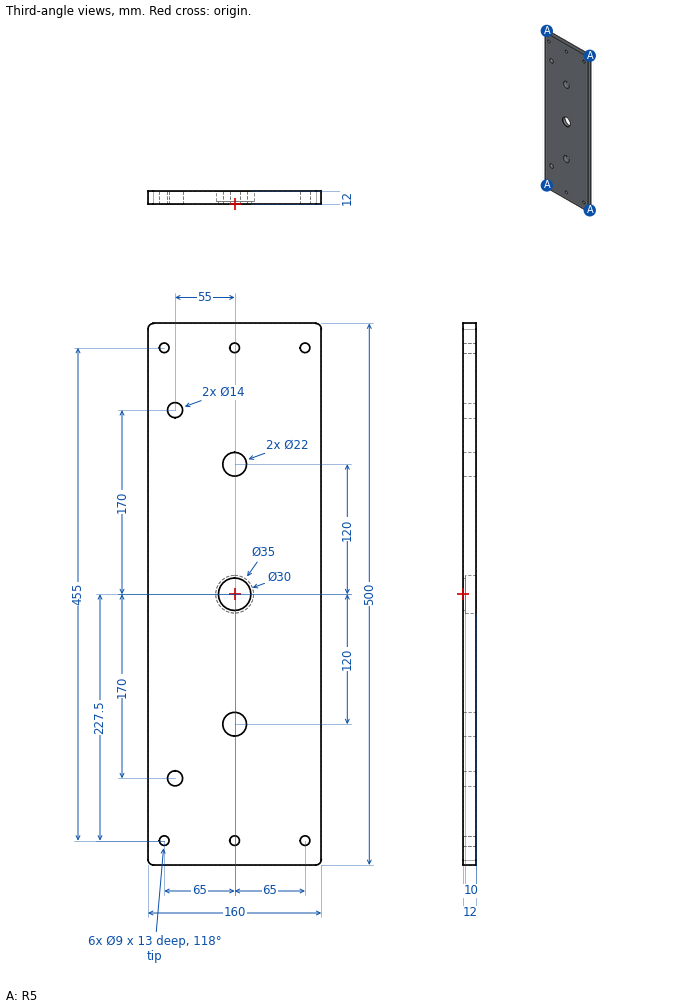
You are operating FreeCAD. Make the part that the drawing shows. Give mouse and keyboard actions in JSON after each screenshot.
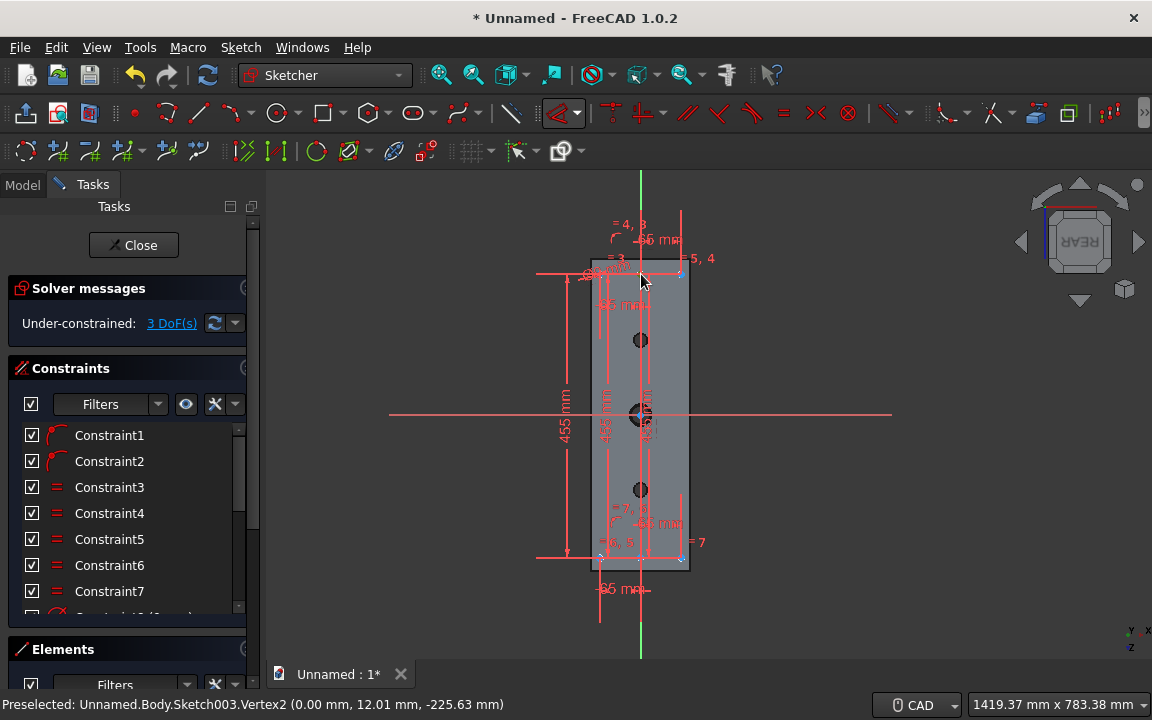
{"action": "left_click", "coordinate": [641, 558]}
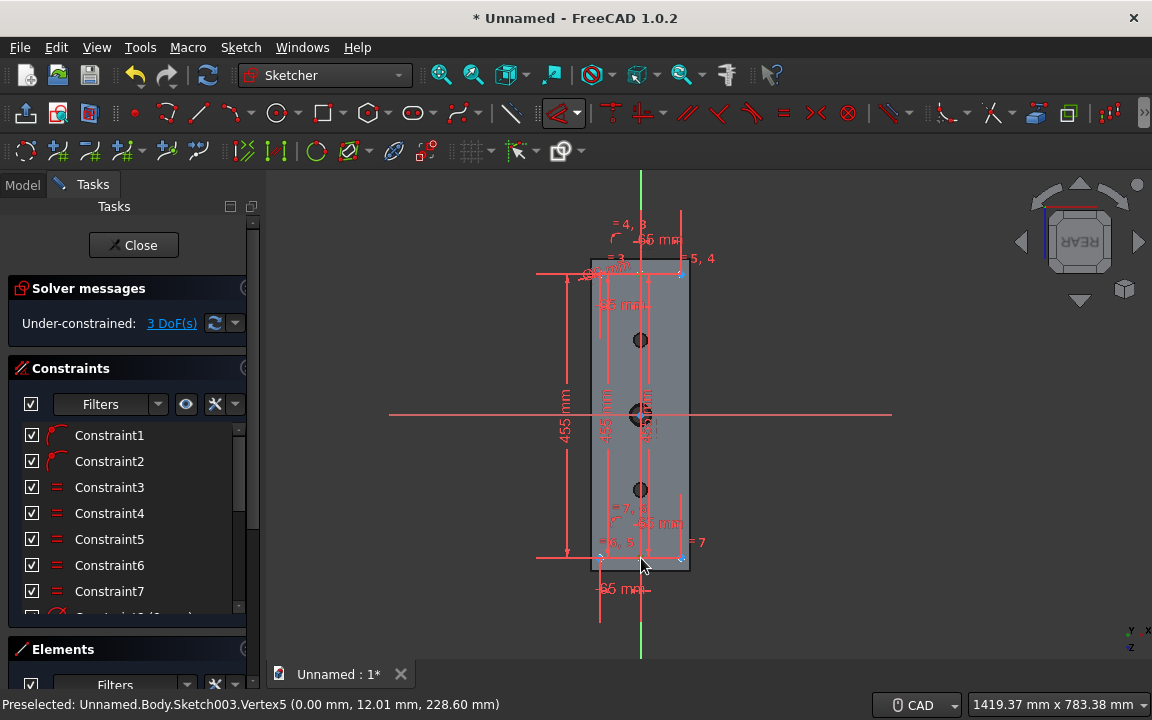
{"action": "left_click", "coordinate": [580, 114]}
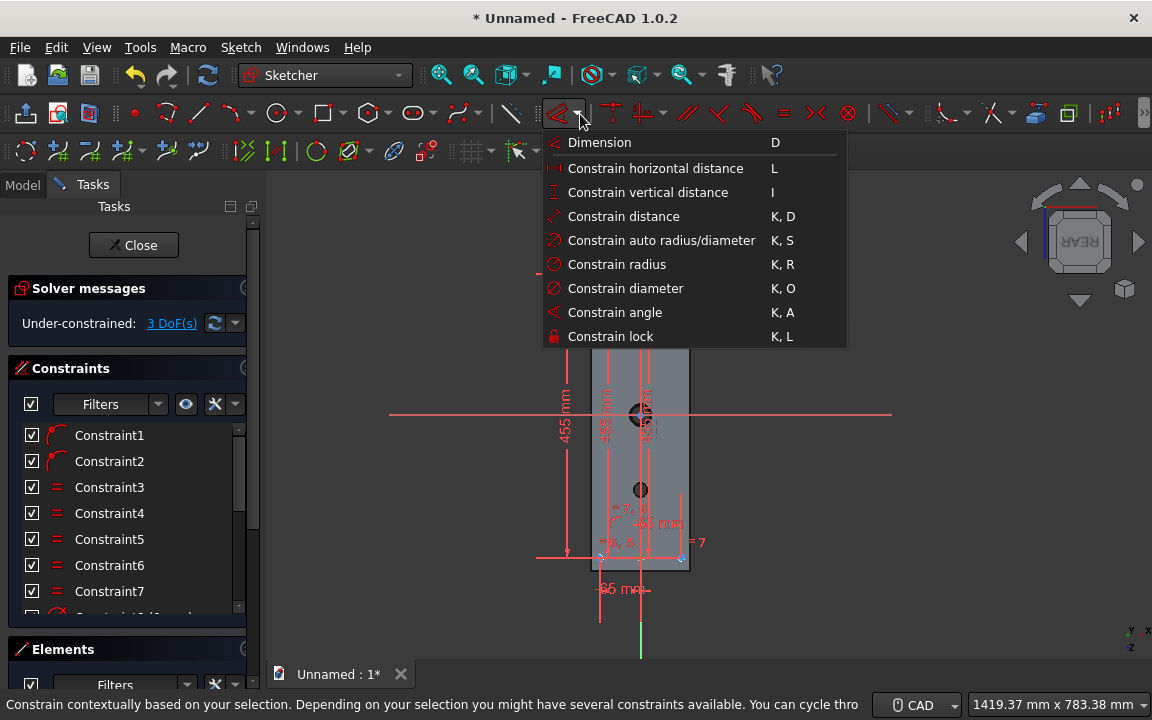
{"action": "left_click", "coordinate": [695, 192]}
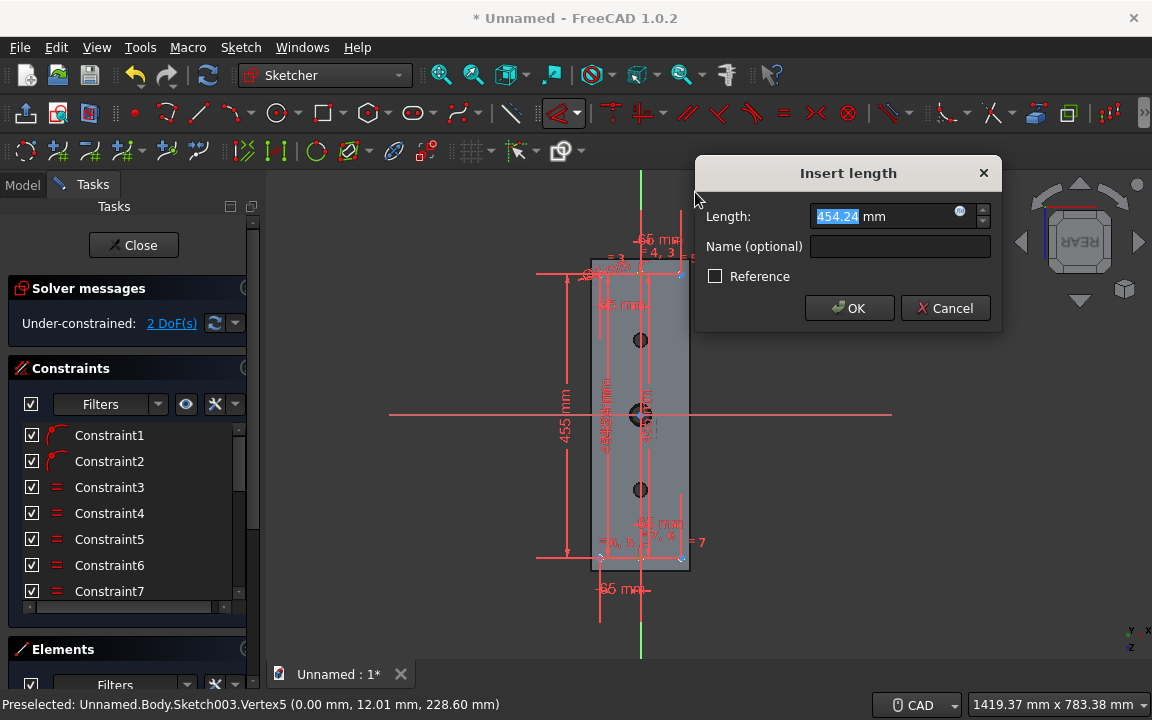
{"action": "type", "text": "455"}
{"action": "key", "text": "Return"}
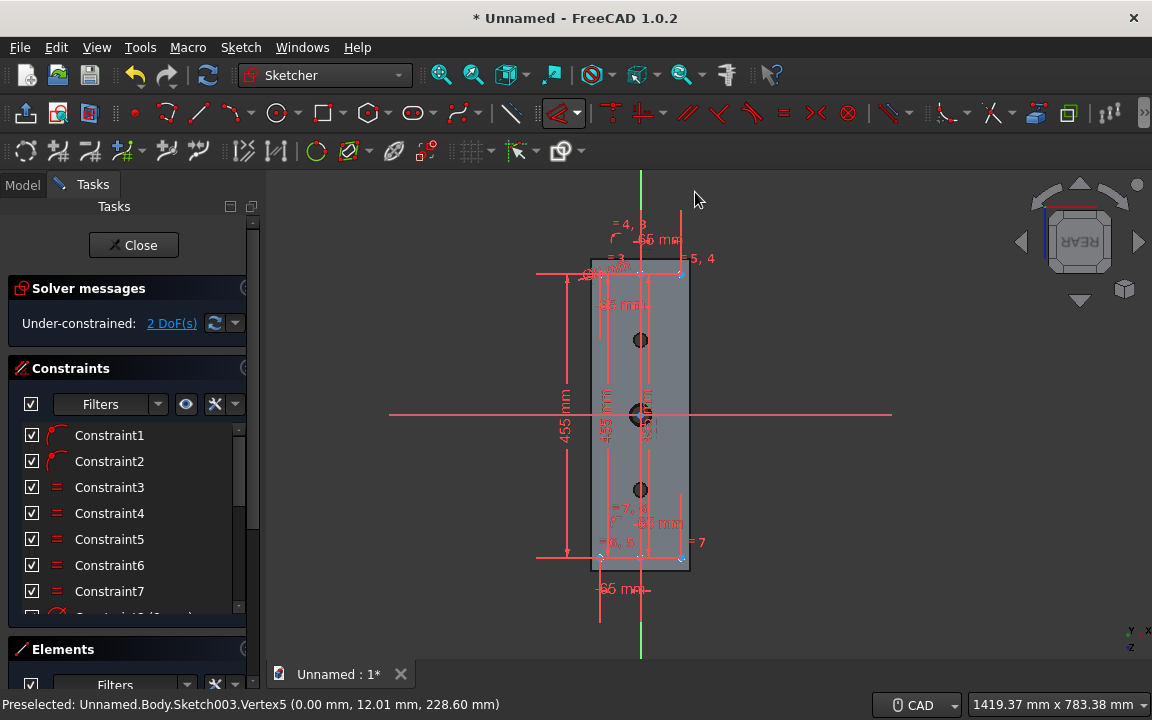
{"action": "left_click", "coordinate": [681, 274]}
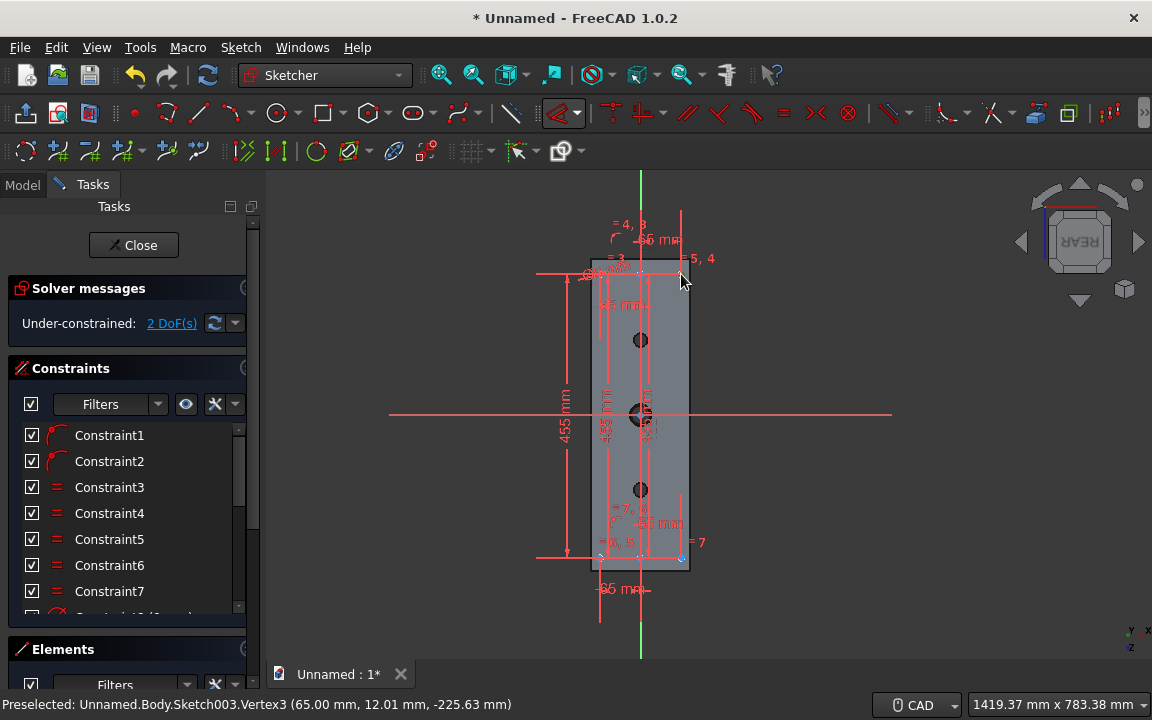
{"action": "left_click", "coordinate": [681, 558]}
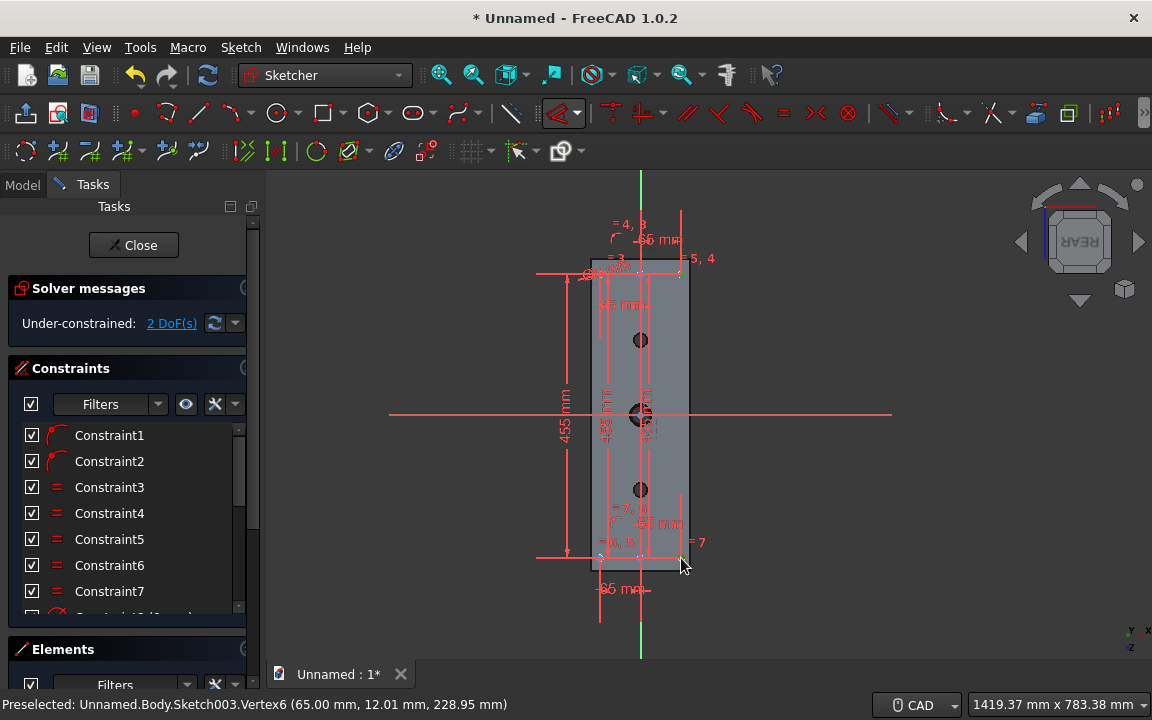
{"action": "left_click", "coordinate": [580, 114]}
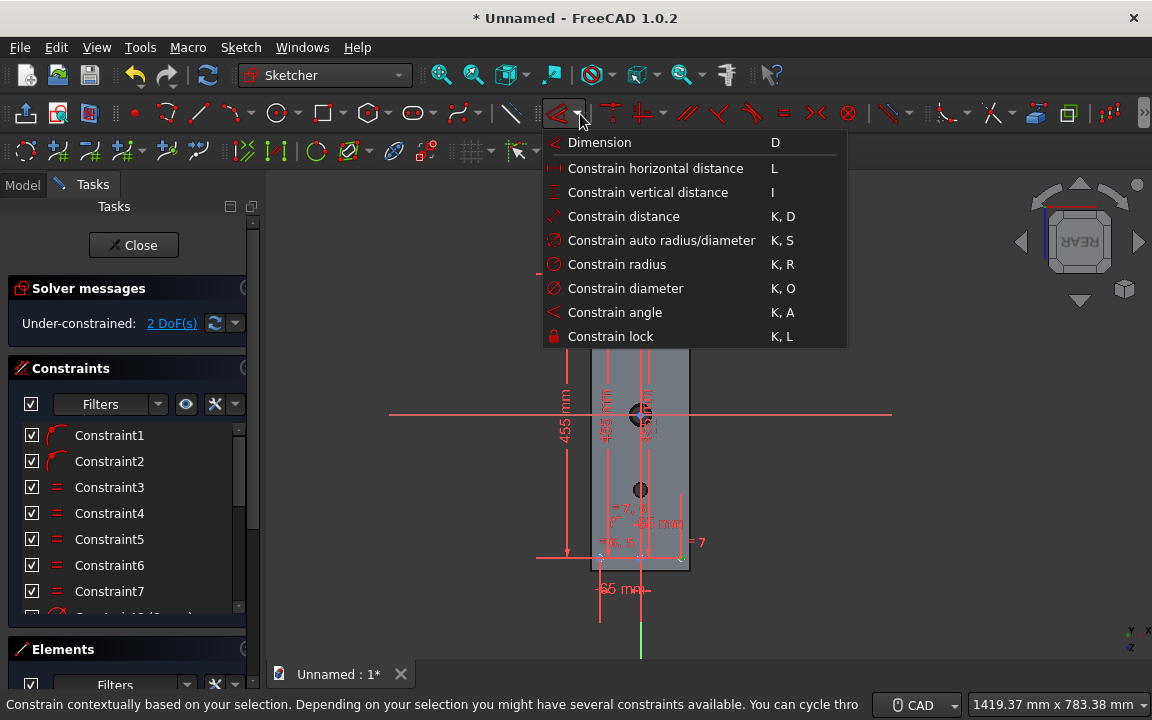
{"action": "left_click", "coordinate": [695, 192]}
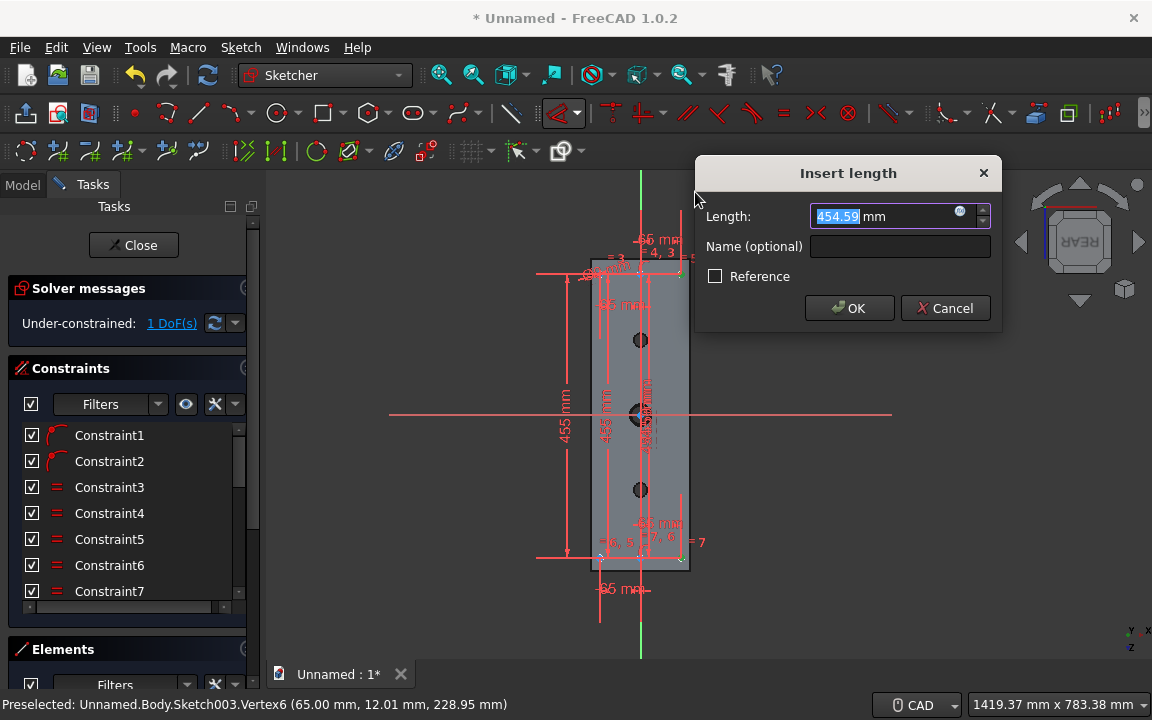
{"action": "type", "text": "455"}
{"action": "key", "text": "Return"}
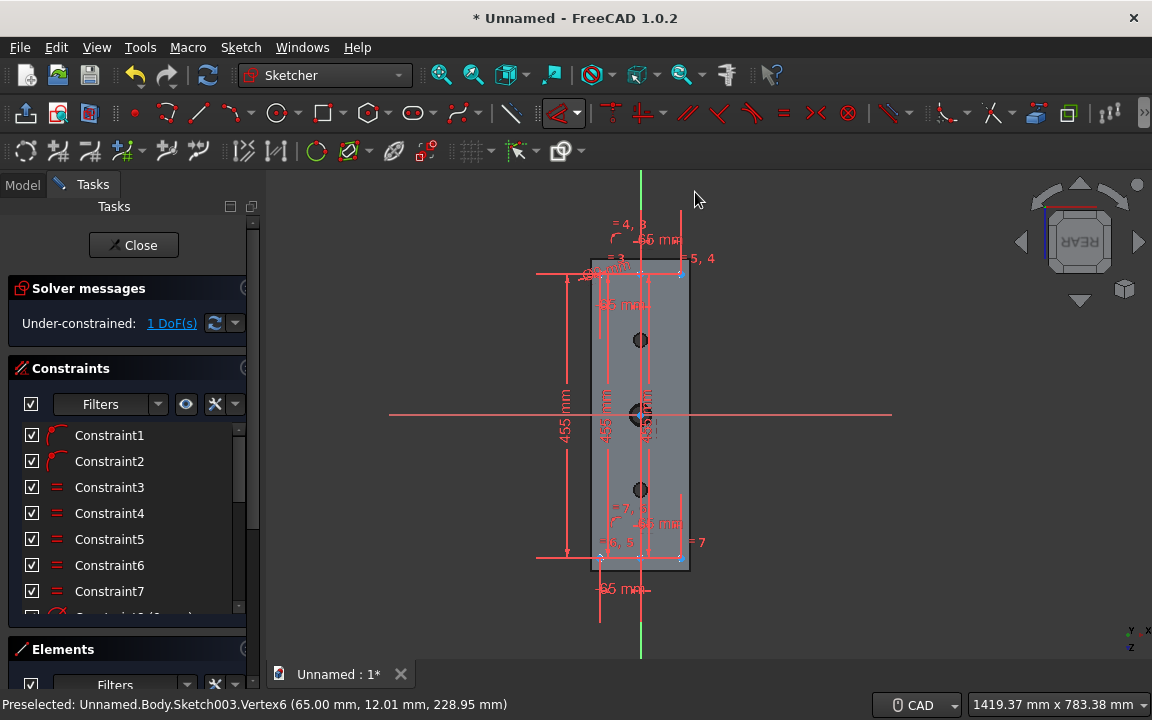
{"action": "left_click", "coordinate": [600, 274]}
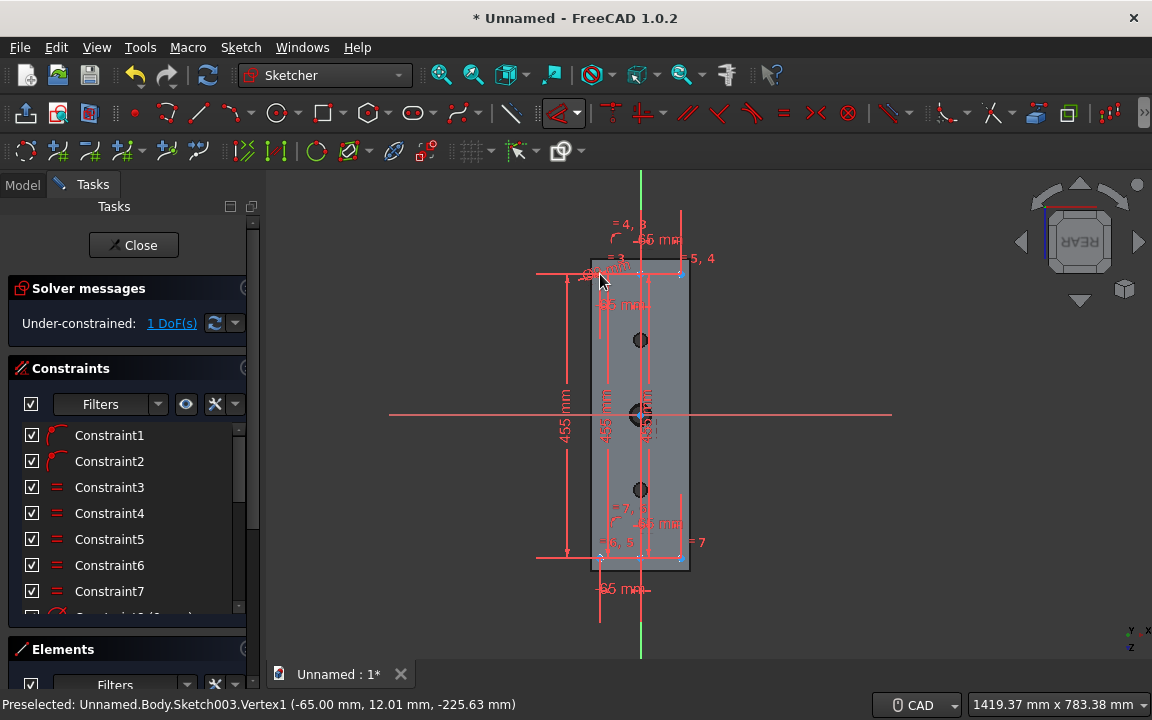
{"action": "left_click", "coordinate": [580, 114]}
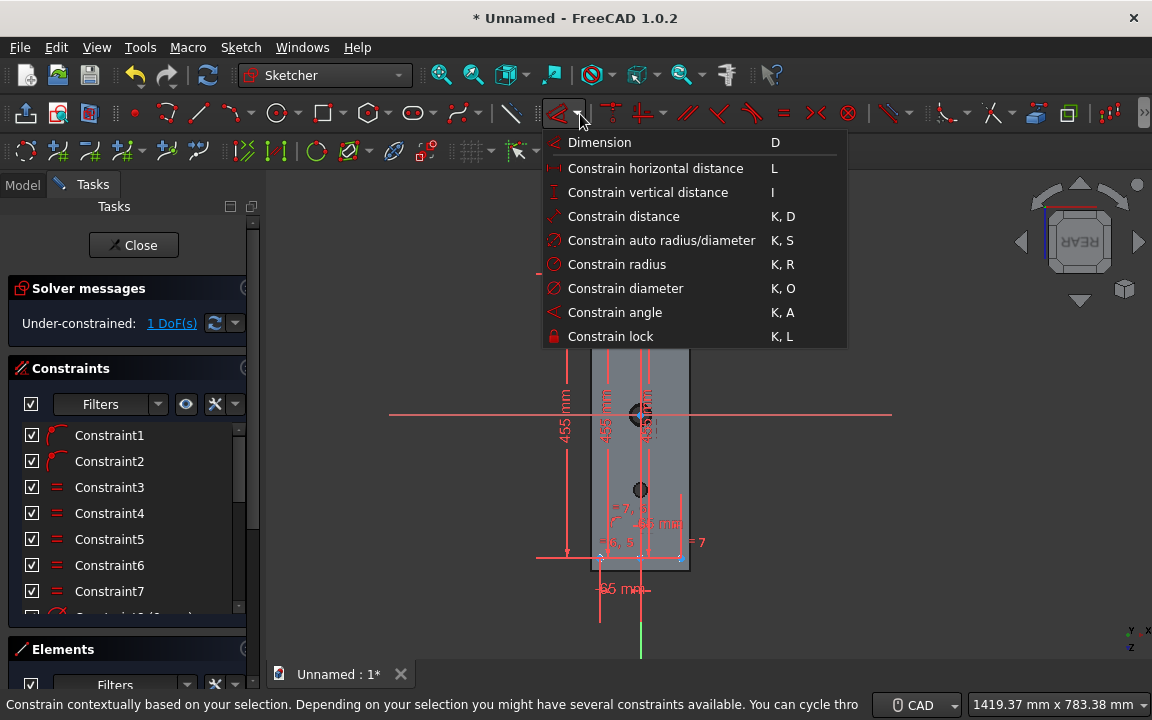
{"action": "left_click", "coordinate": [695, 192]}